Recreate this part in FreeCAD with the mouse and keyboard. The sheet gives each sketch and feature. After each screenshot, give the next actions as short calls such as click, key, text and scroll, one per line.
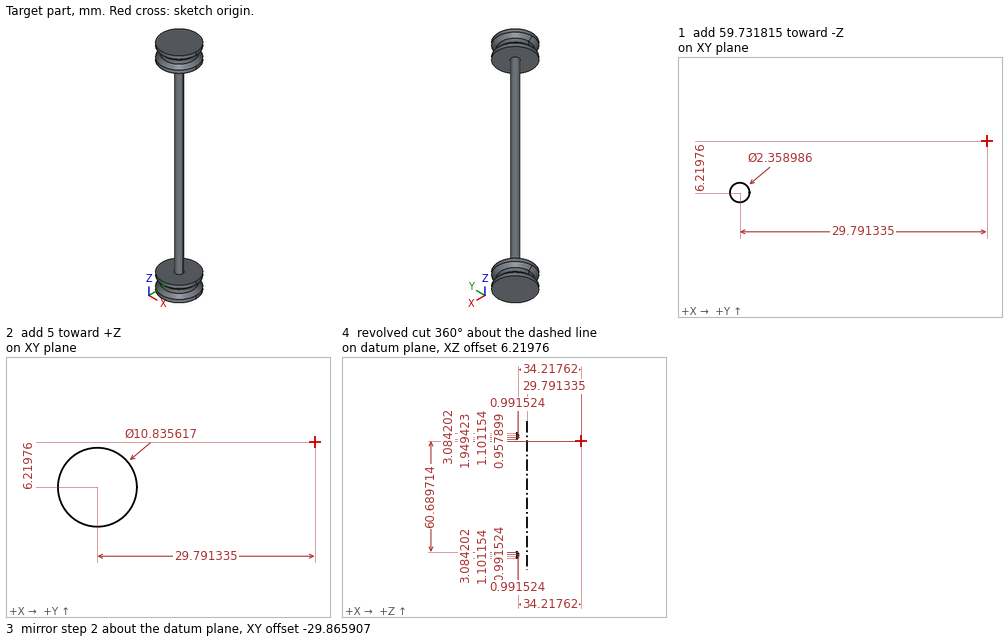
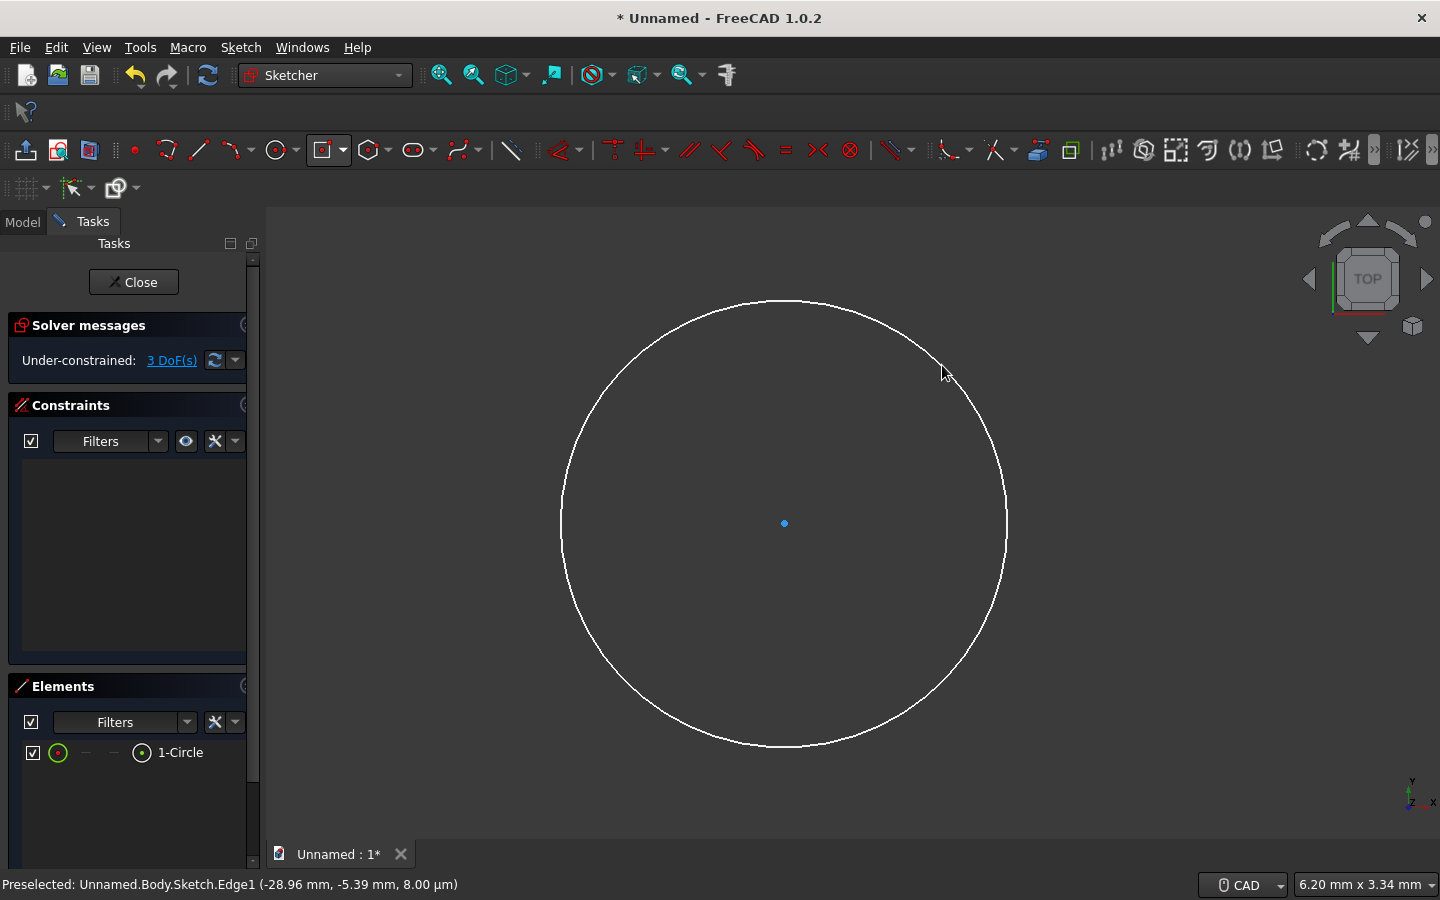
click(942, 366)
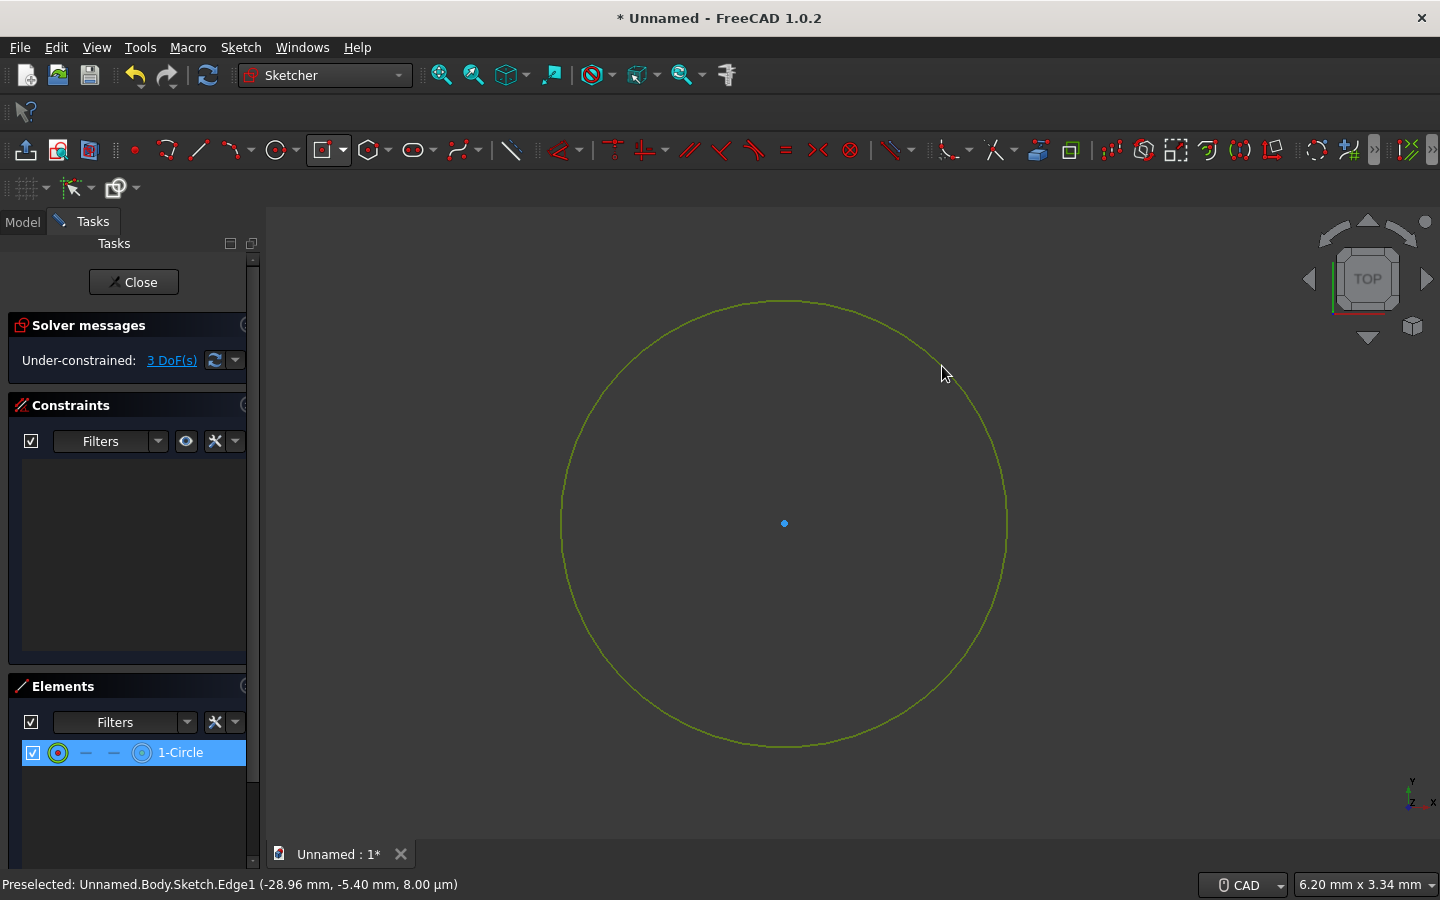
click(582, 150)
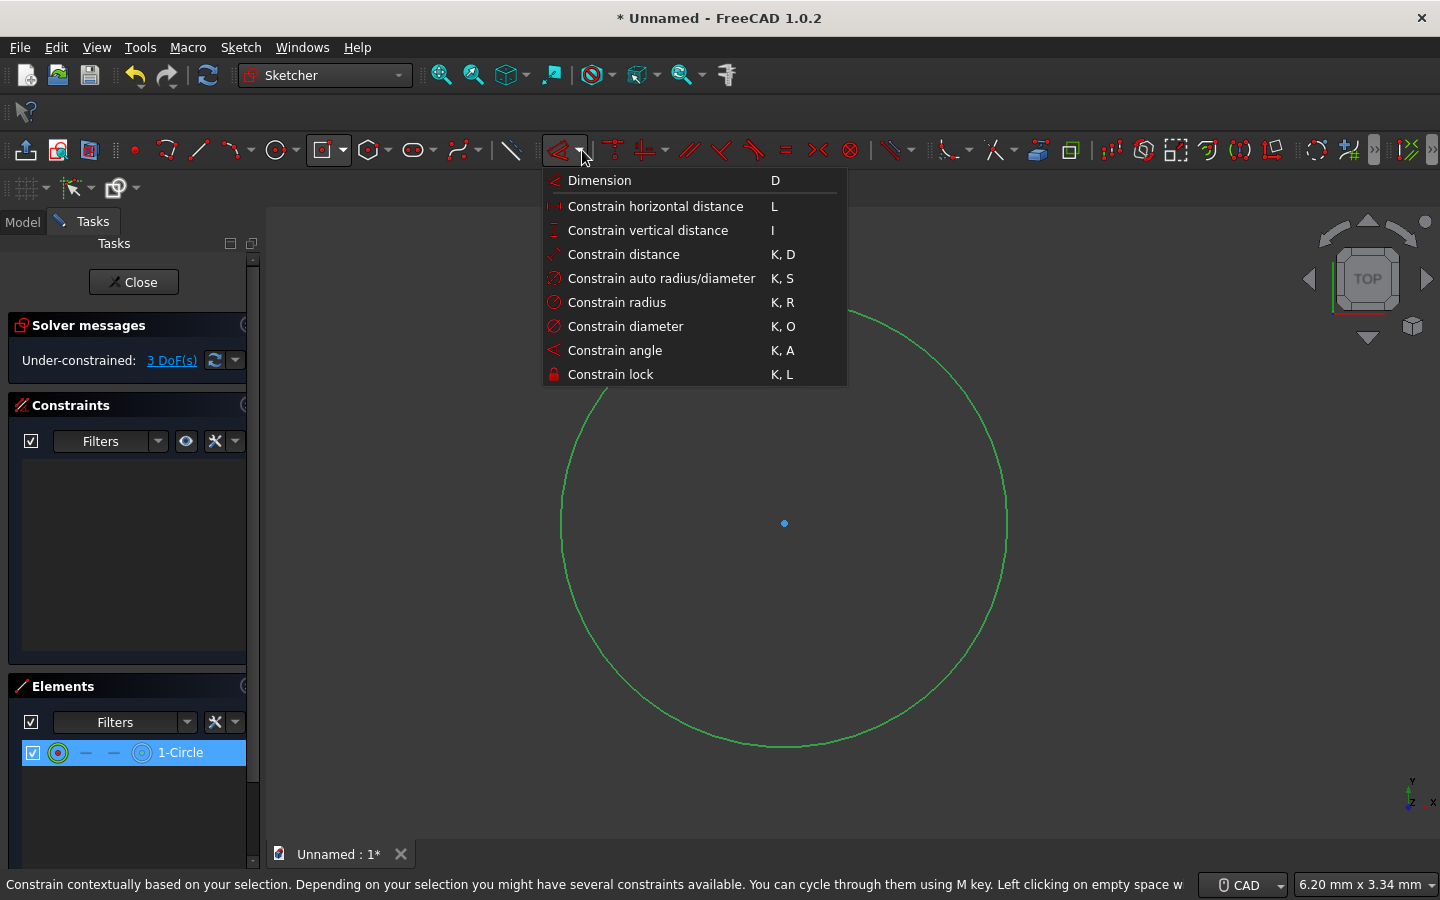
click(695, 326)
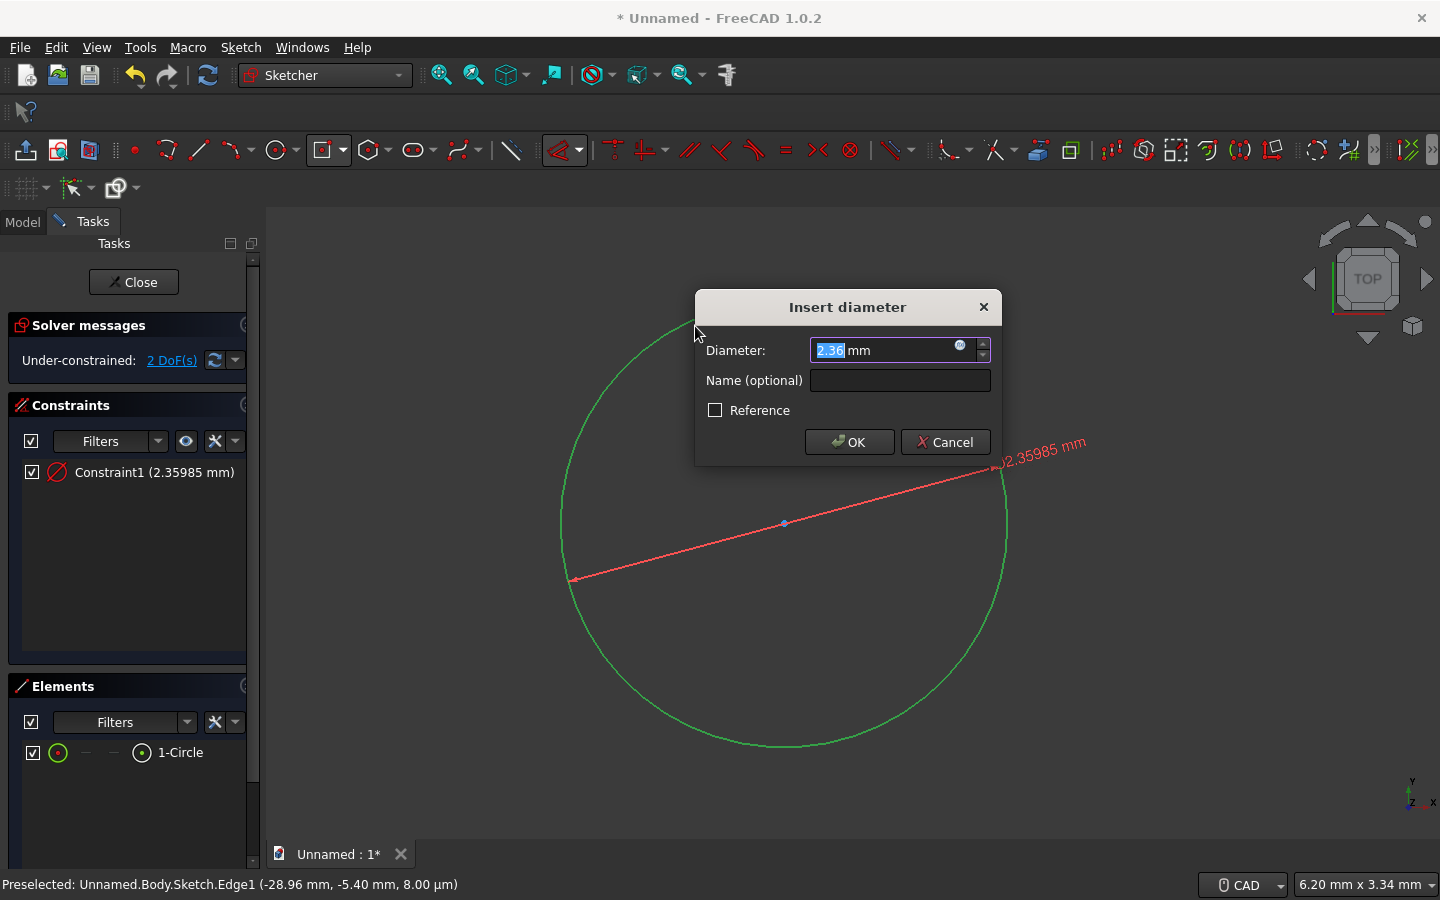
text(2.358986)
key(Return)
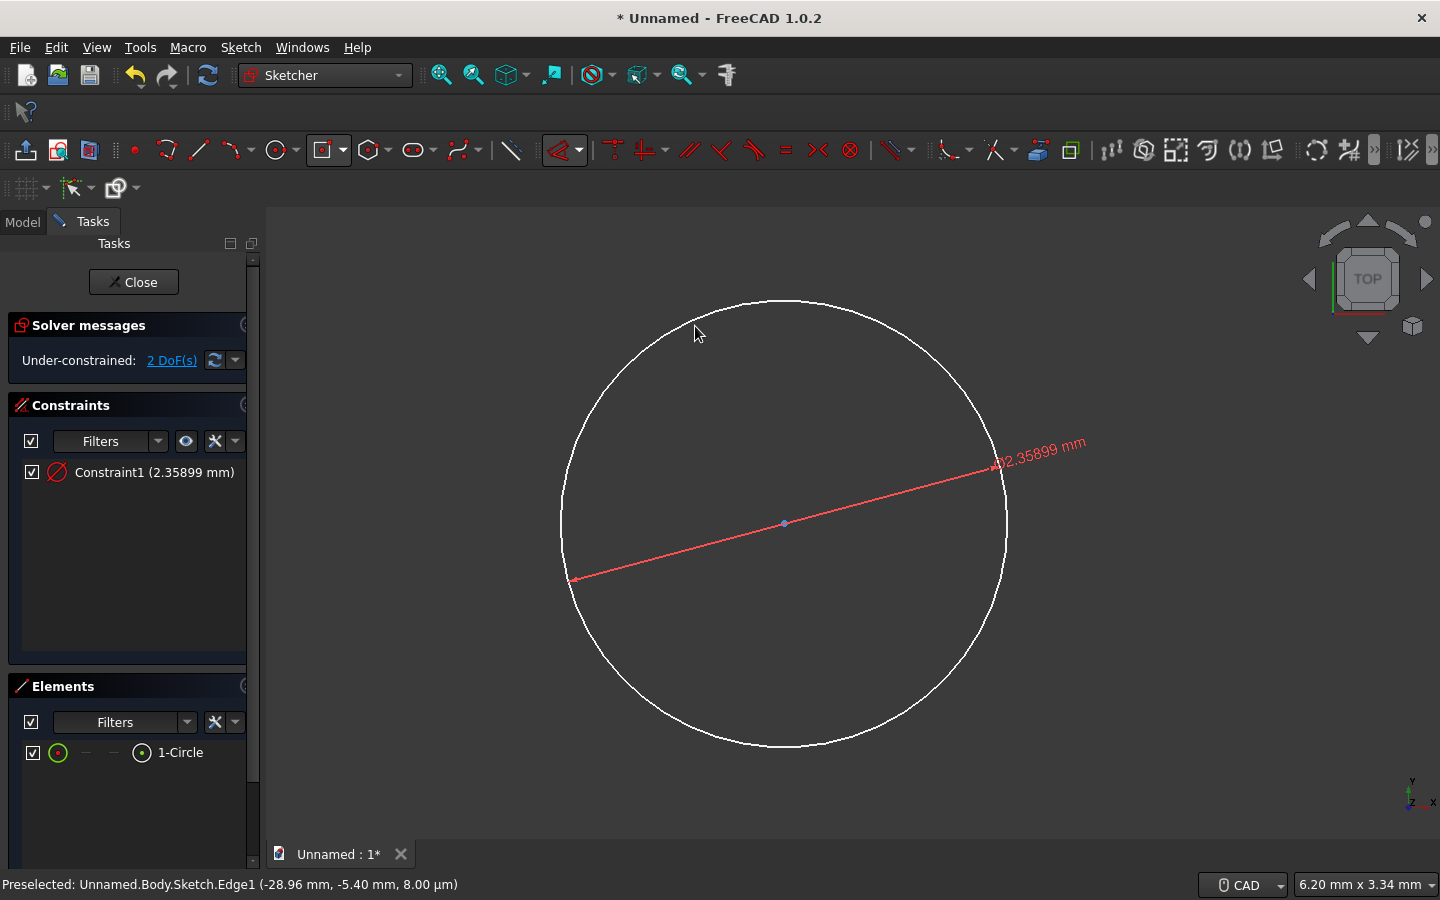
click(784, 524)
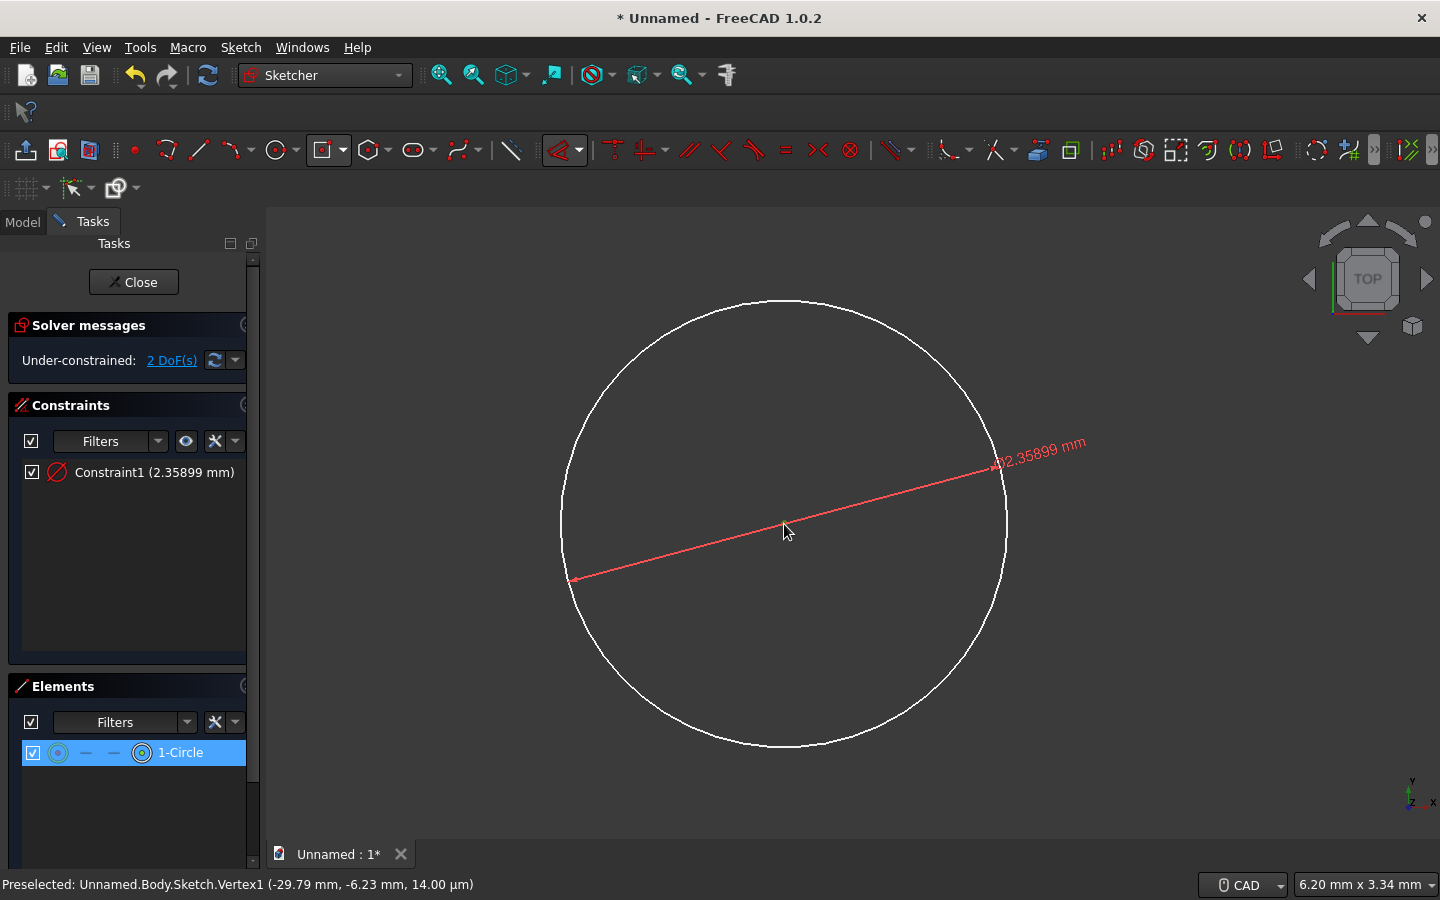
key(i)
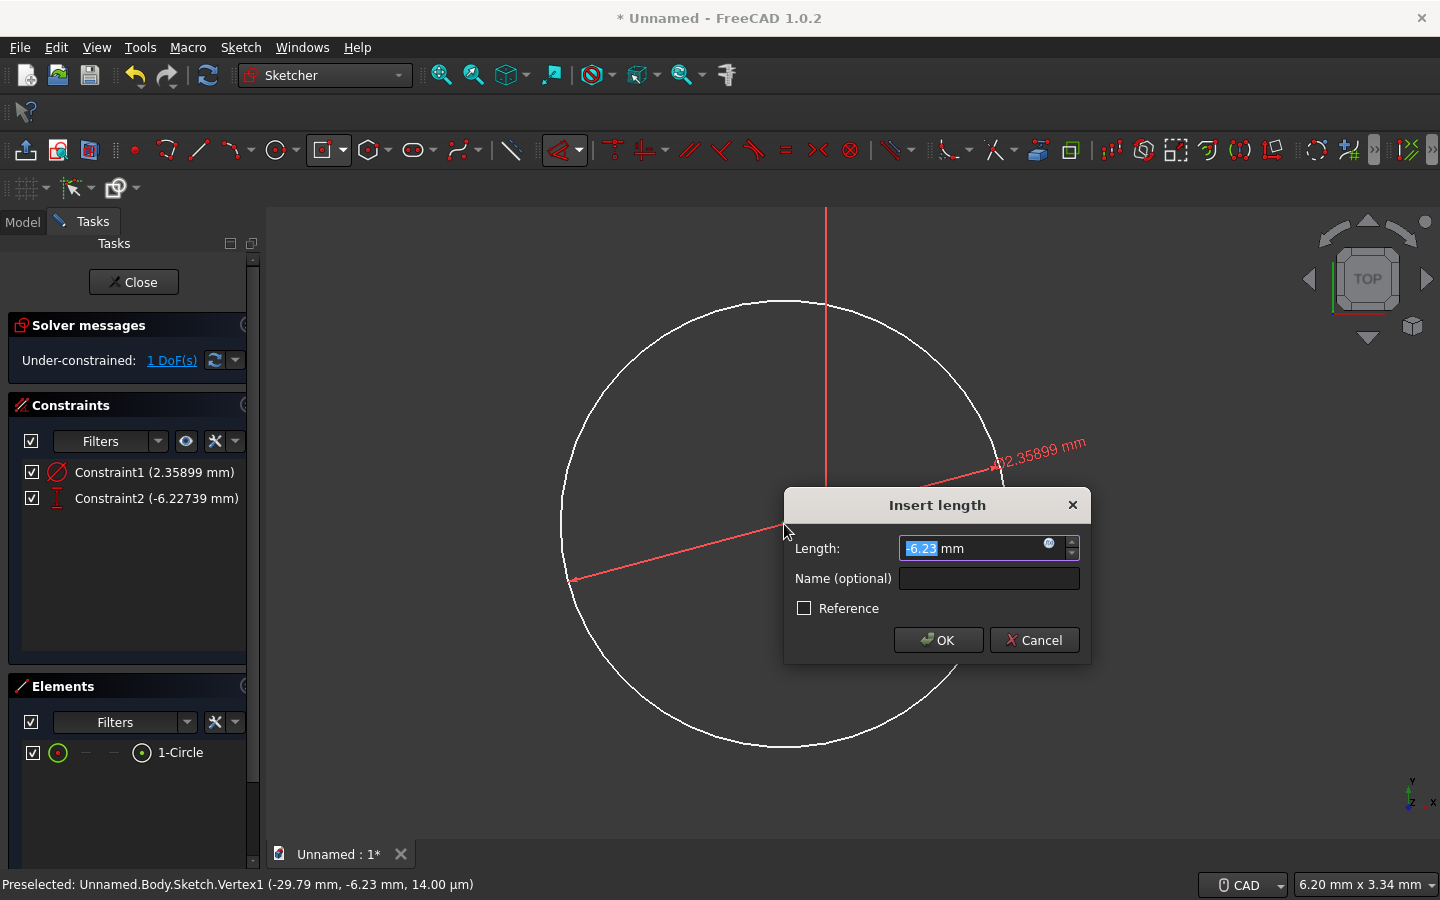
text(-6.21976)
key(Return)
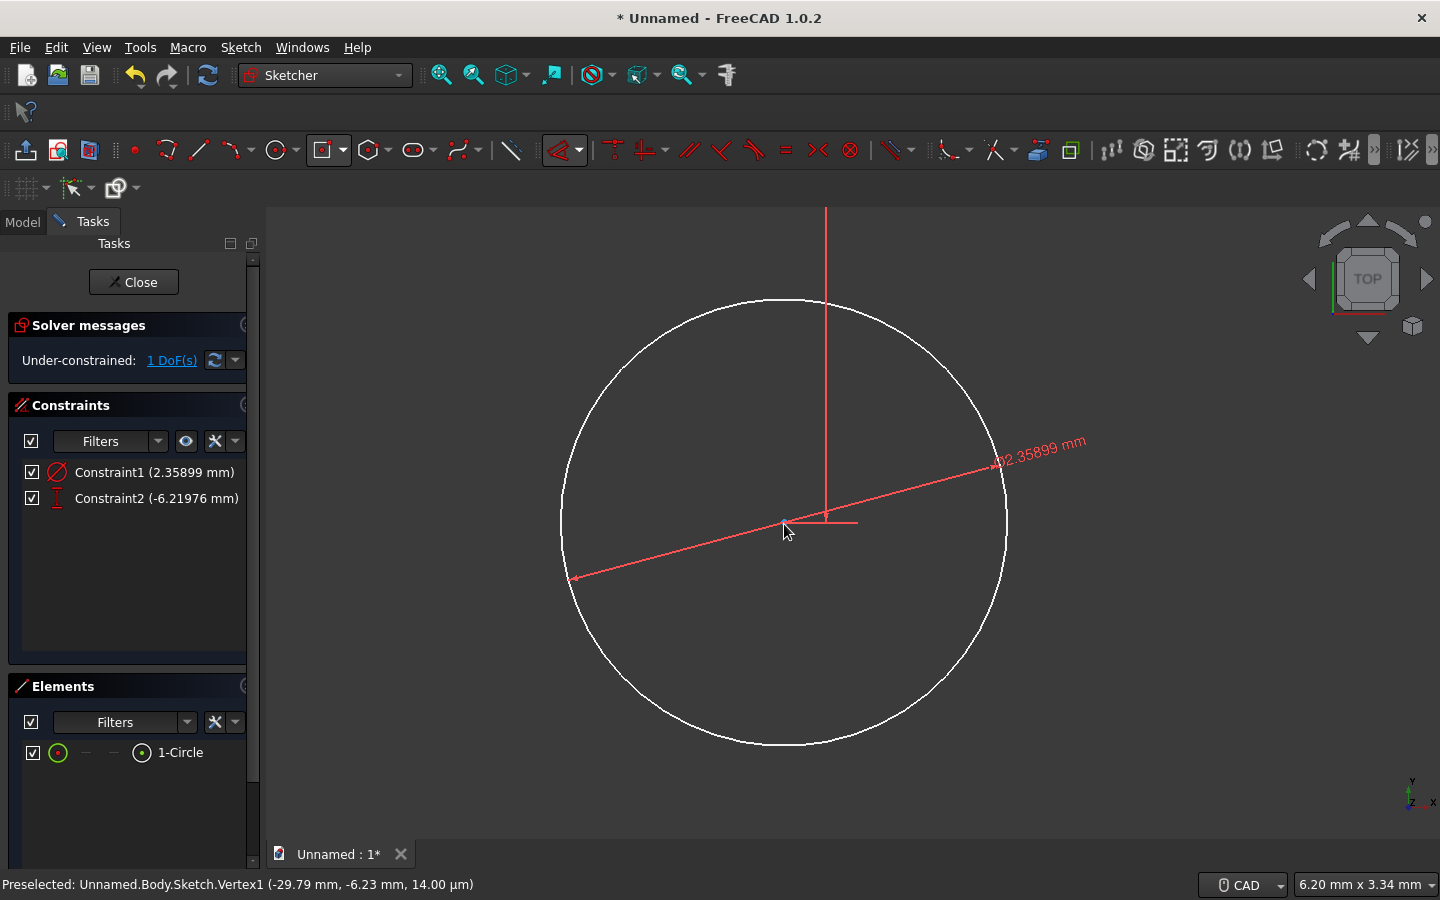
click(784, 523)